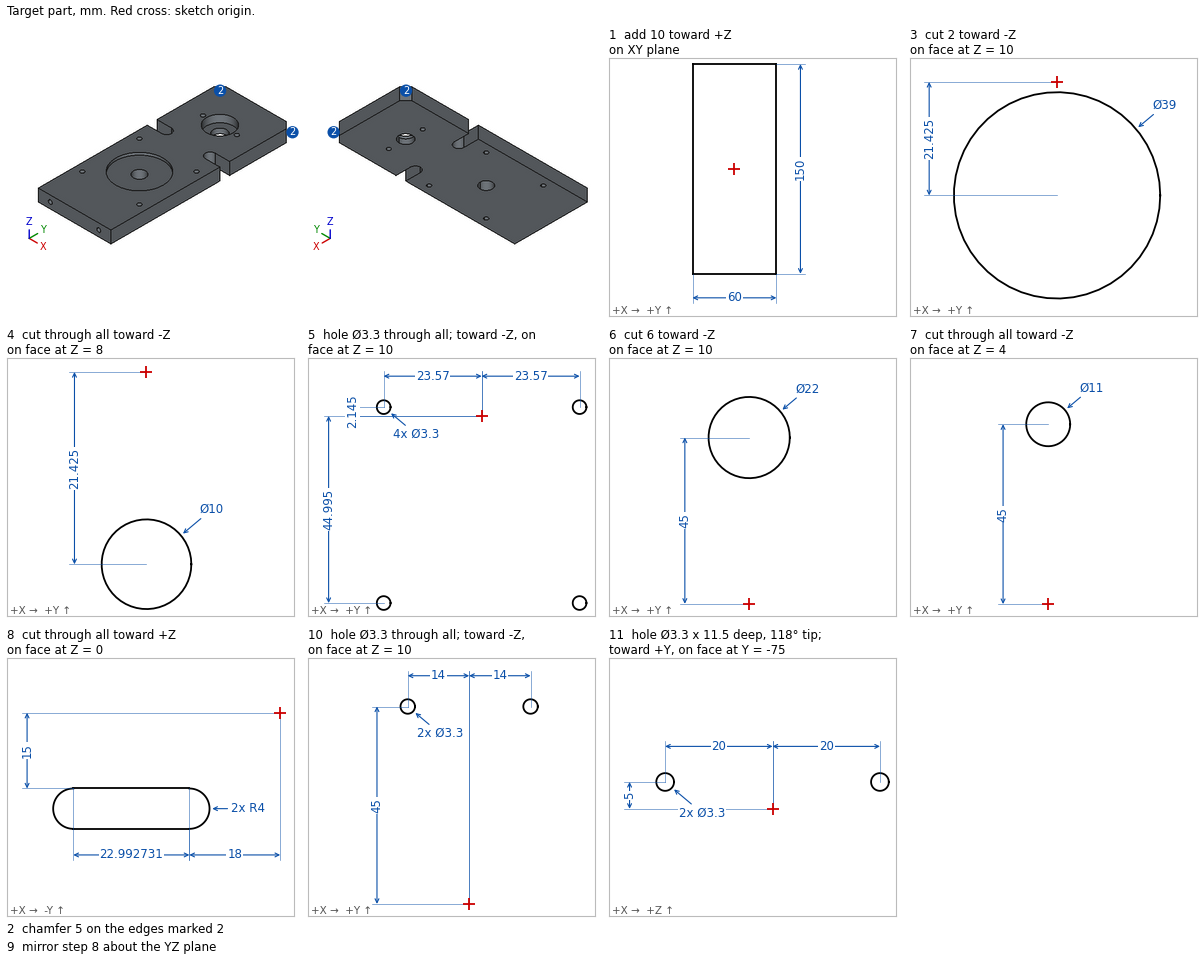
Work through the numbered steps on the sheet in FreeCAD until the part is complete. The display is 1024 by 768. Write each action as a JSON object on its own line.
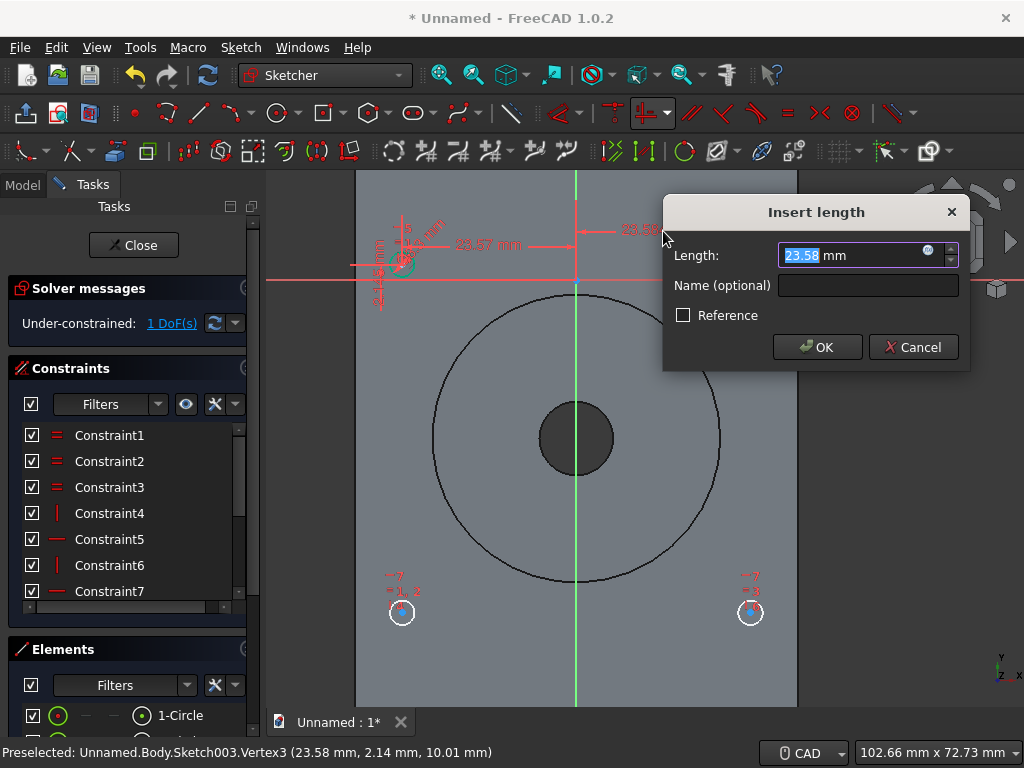
{"action": "type", "text": "23.57"}
{"action": "key", "text": "Return"}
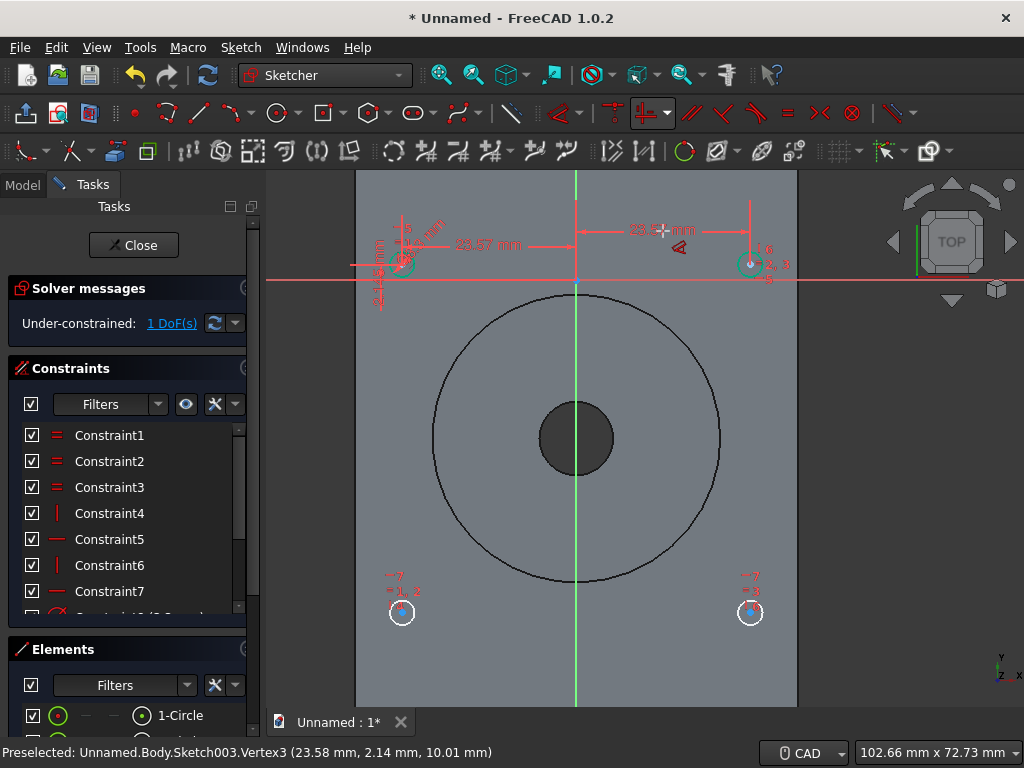
{"action": "left_click", "coordinate": [402, 613]}
{"action": "left_click", "coordinate": [368, 447]}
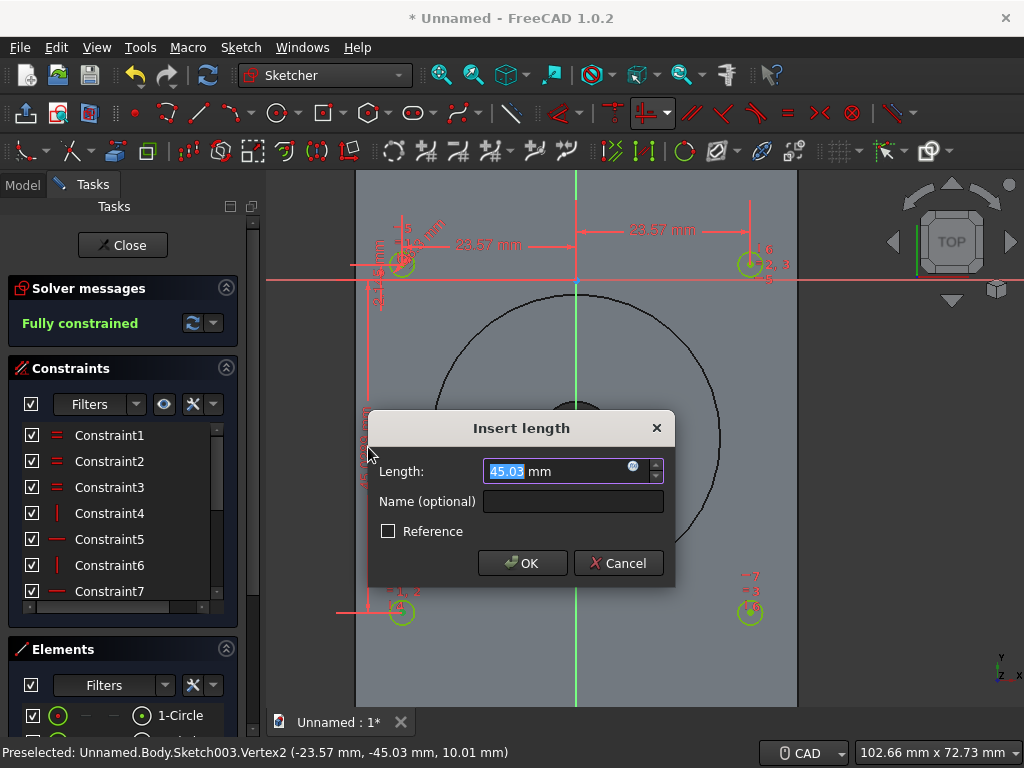
{"action": "type", "text": "44.995"}
{"action": "key", "text": "Return"}
{"action": "key", "text": "Escape"}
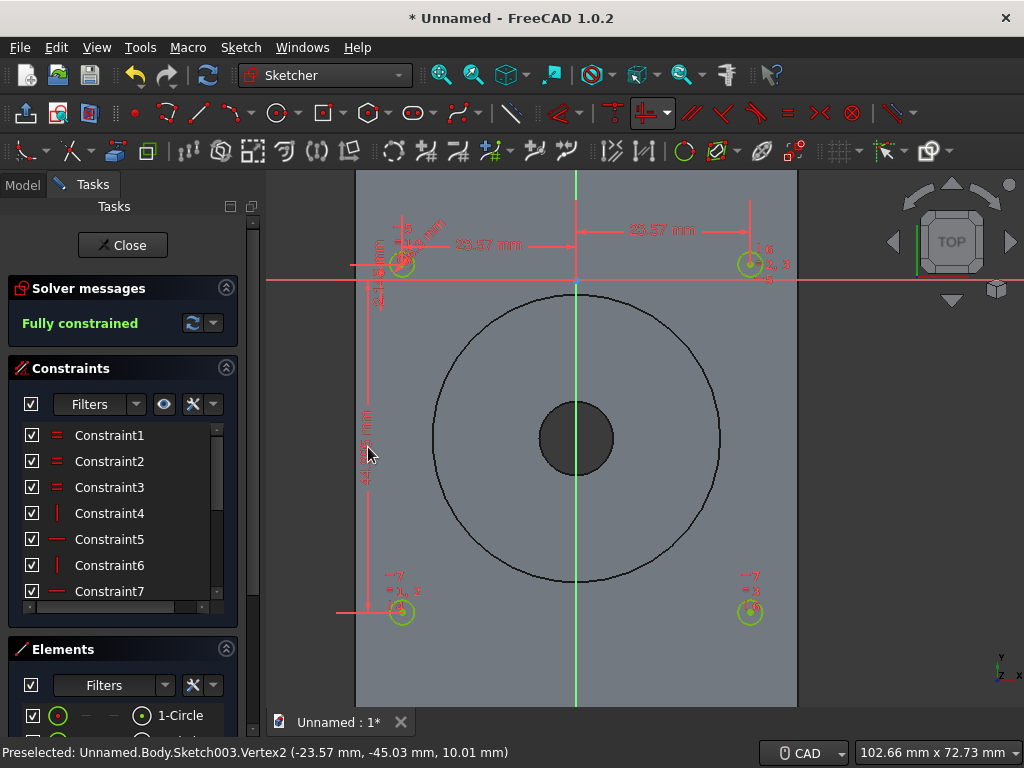
{"action": "left_click", "coordinate": [123, 245]}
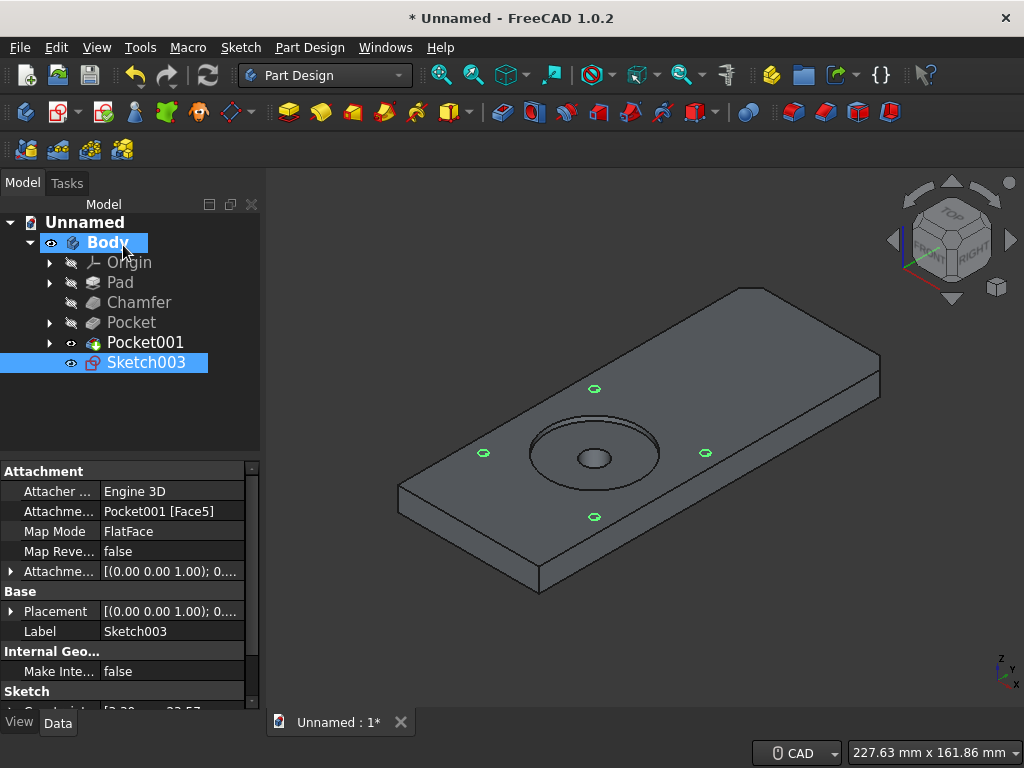
{"action": "left_click", "coordinate": [536, 112]}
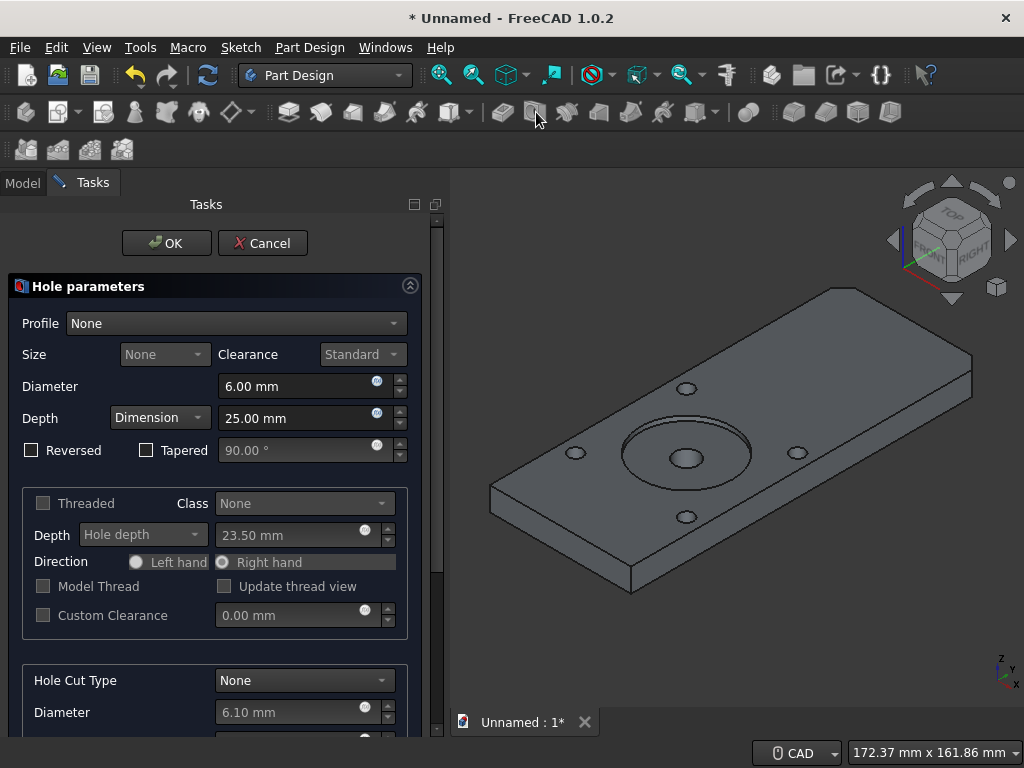
{"action": "triple_click", "coordinate": [305, 386]}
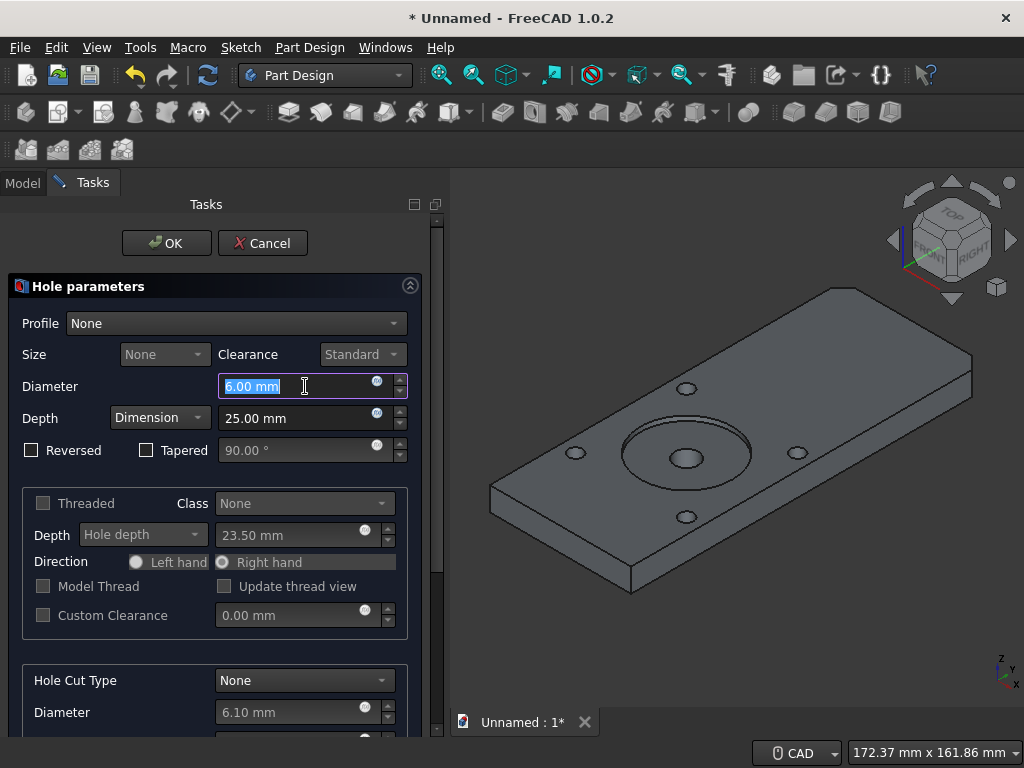
{"action": "type", "text": "3.3"}
{"action": "key", "text": "Tab"}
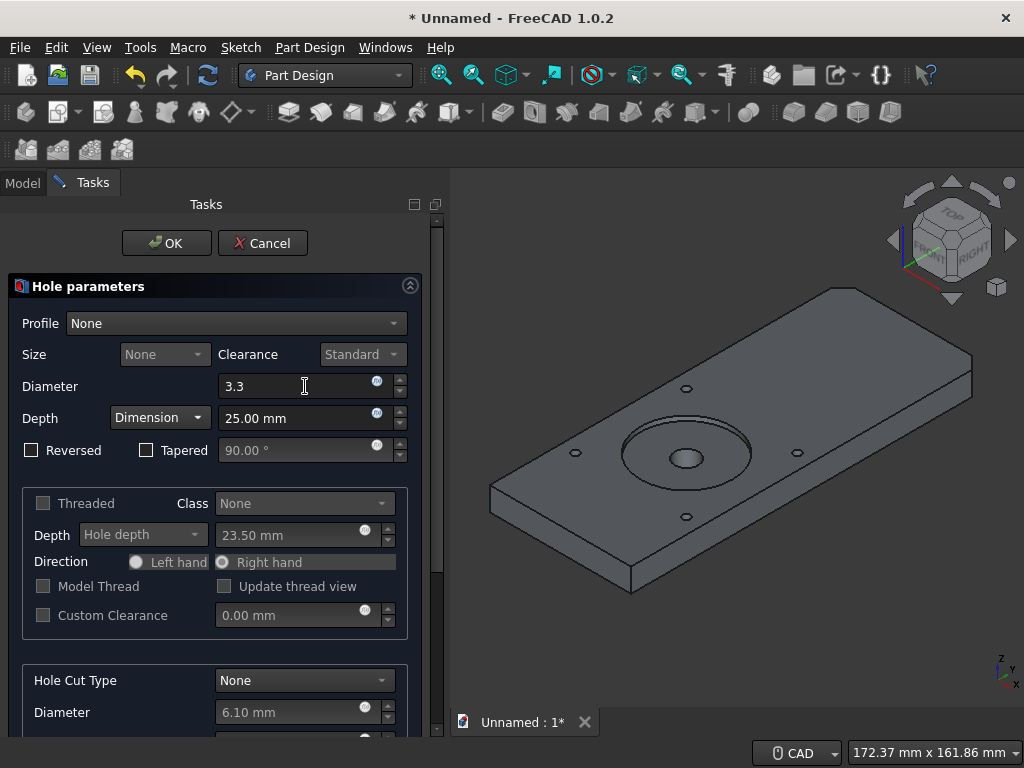
{"action": "left_click", "coordinate": [161, 418]}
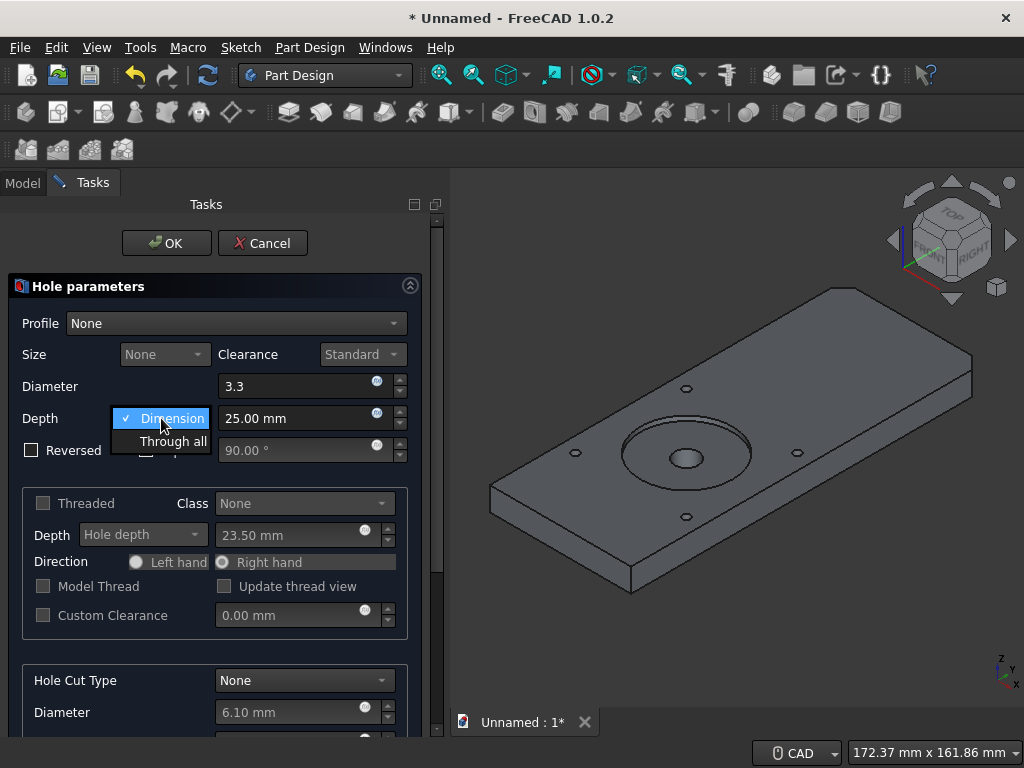
{"action": "left_click", "coordinate": [160, 442]}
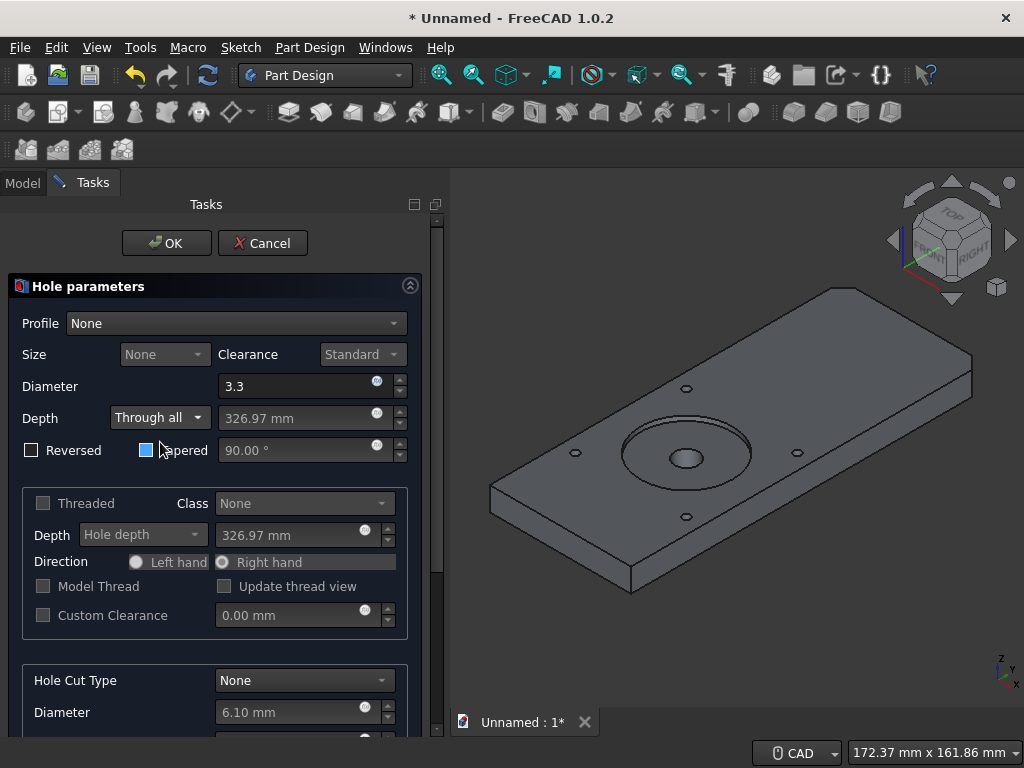
{"action": "left_click", "coordinate": [167, 243]}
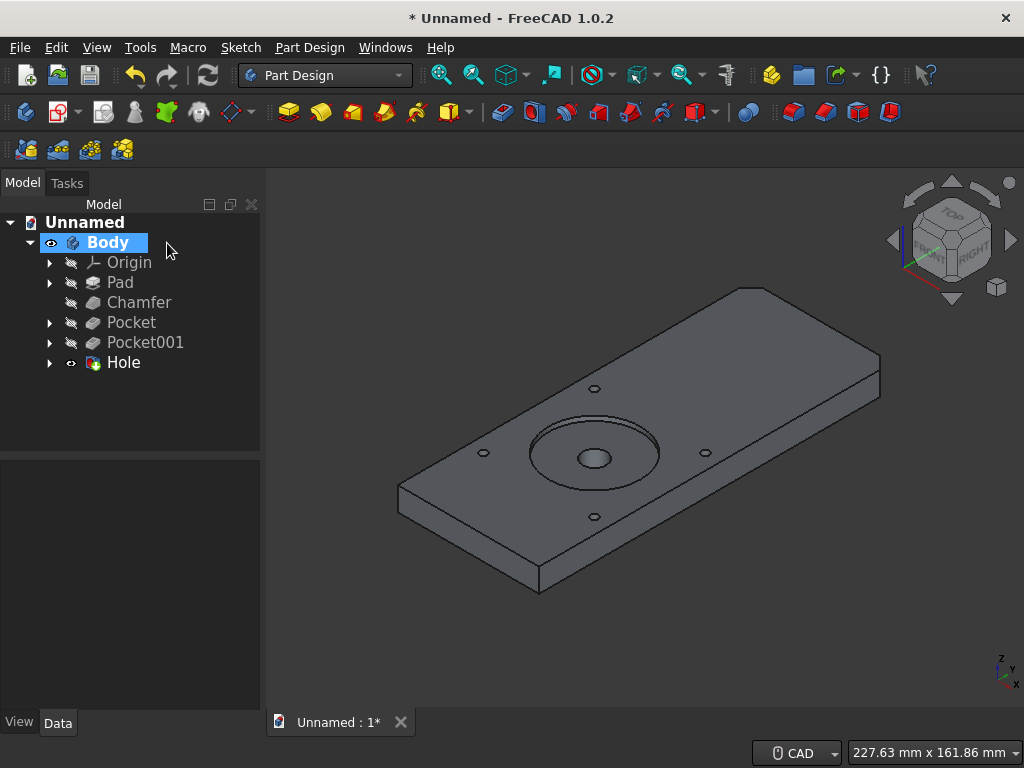
{"action": "left_click", "coordinate": [746, 365]}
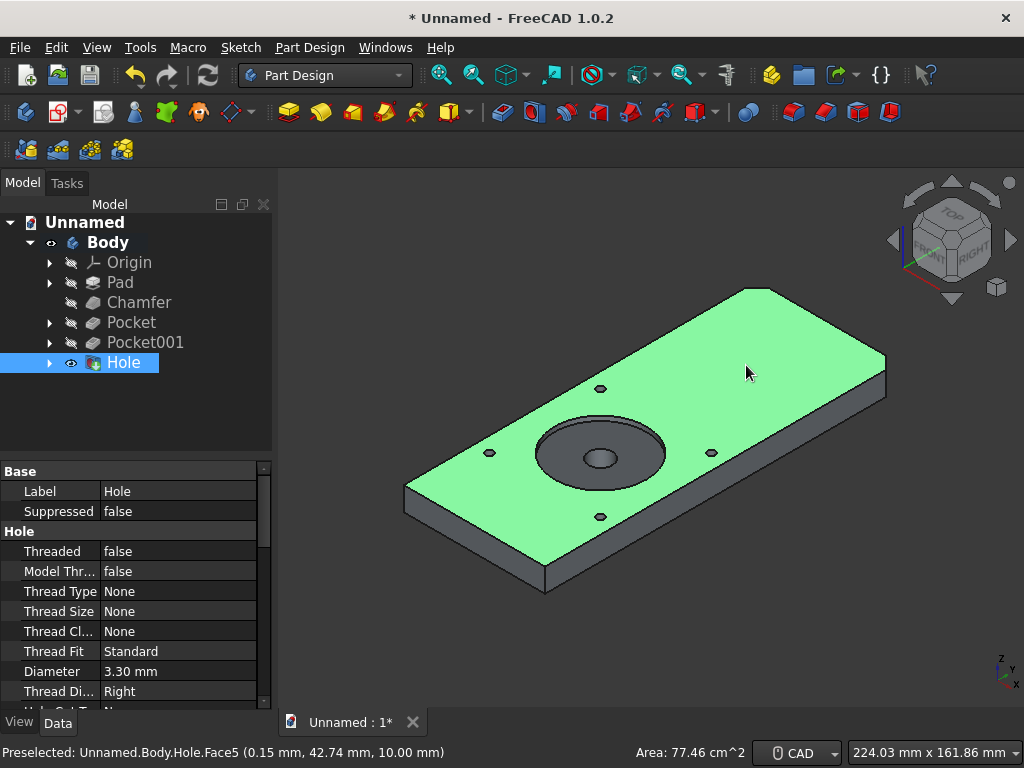
{"action": "left_click", "coordinate": [58, 112]}